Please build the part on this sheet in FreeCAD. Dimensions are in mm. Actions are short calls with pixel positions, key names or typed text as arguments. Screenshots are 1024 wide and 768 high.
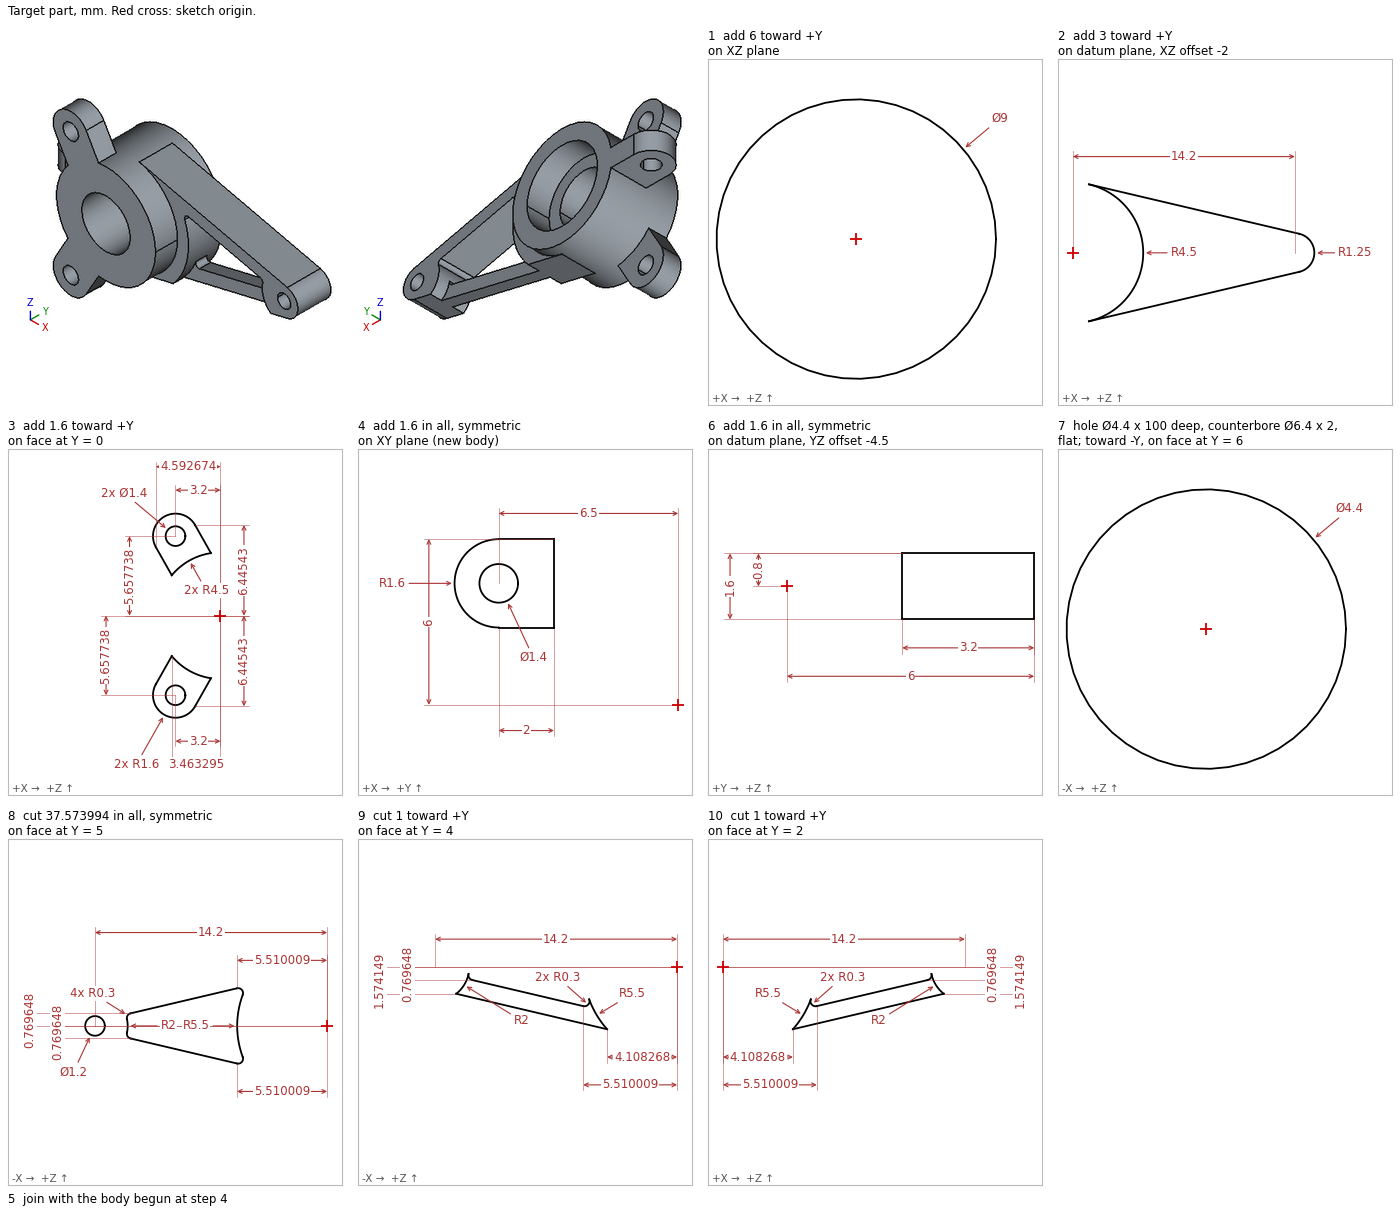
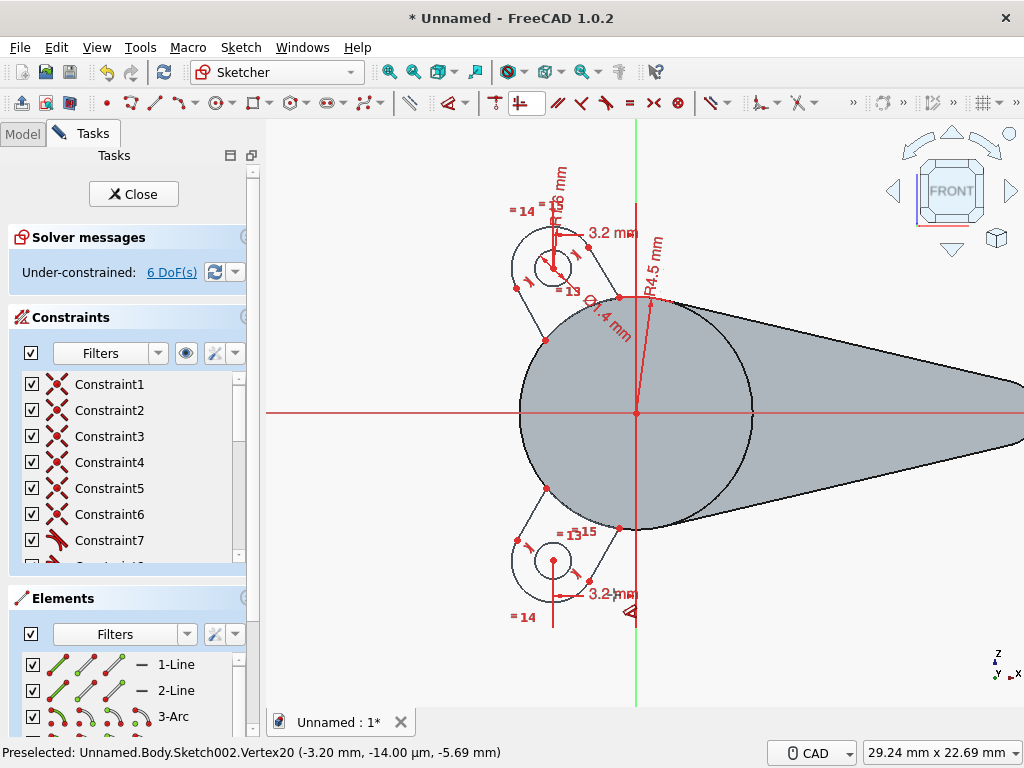
click(589, 247)
click(670, 292)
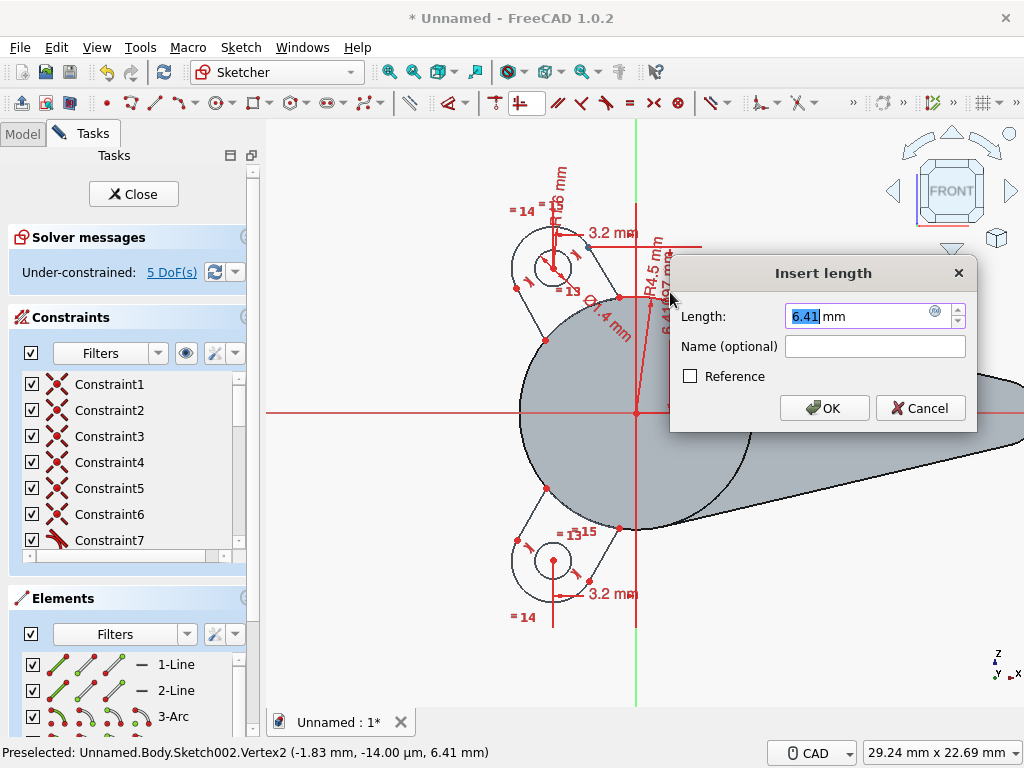
text(6.44543)
key(Return)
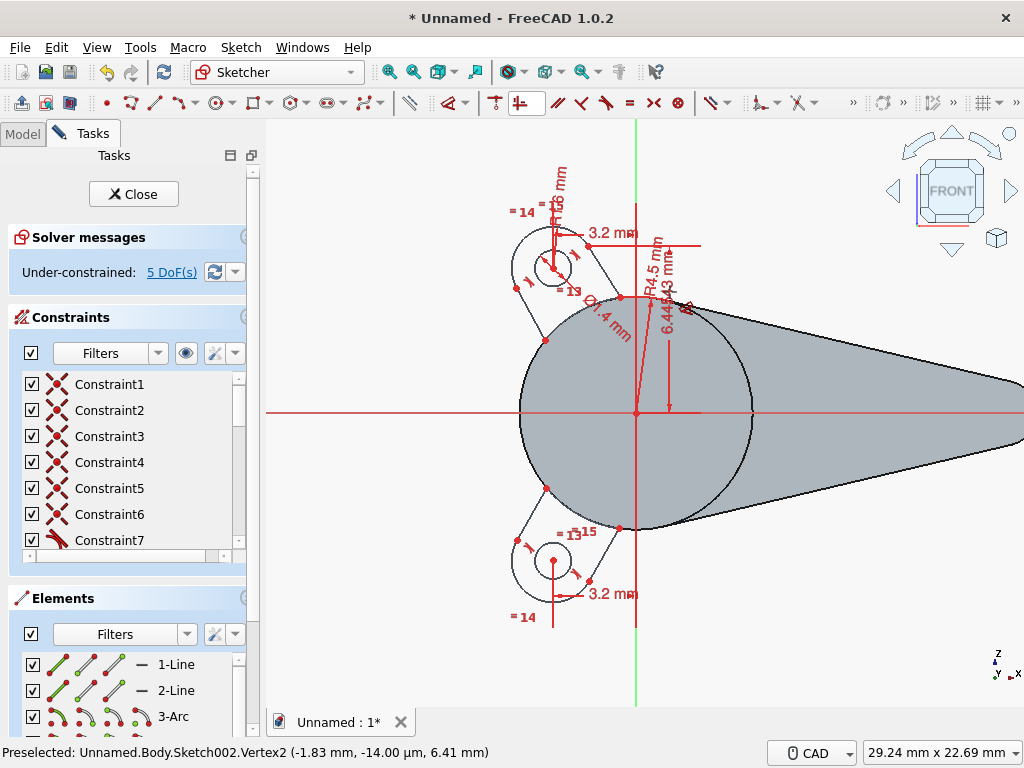
click(589, 581)
click(670, 497)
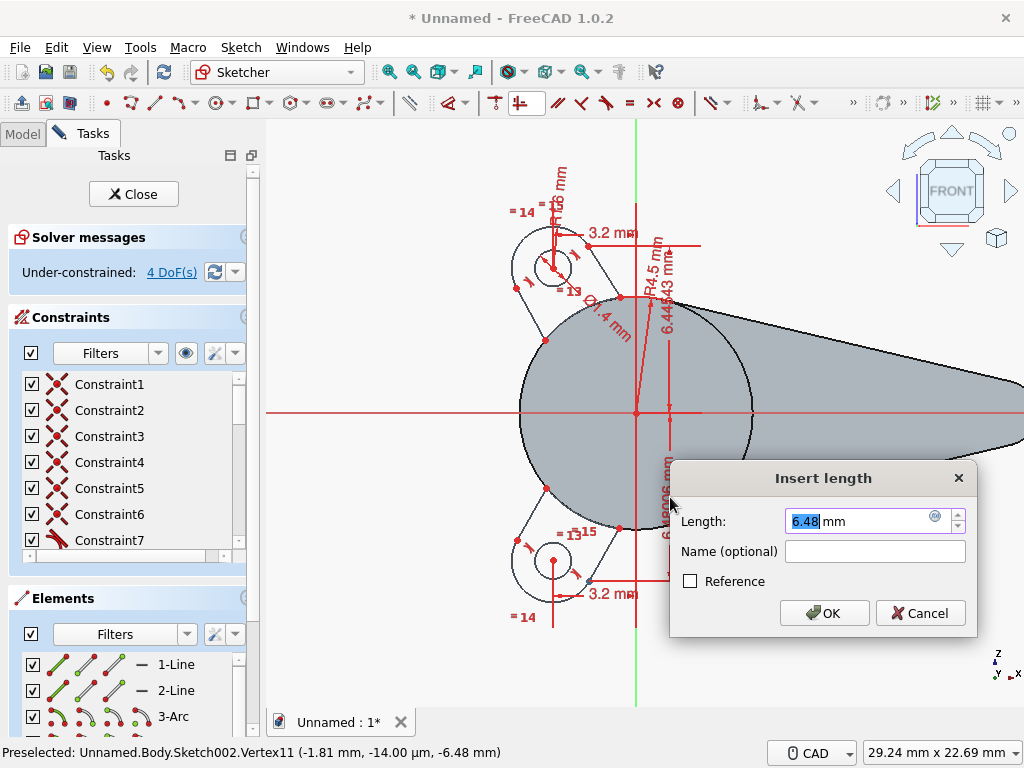
text(6.44543)
key(Return)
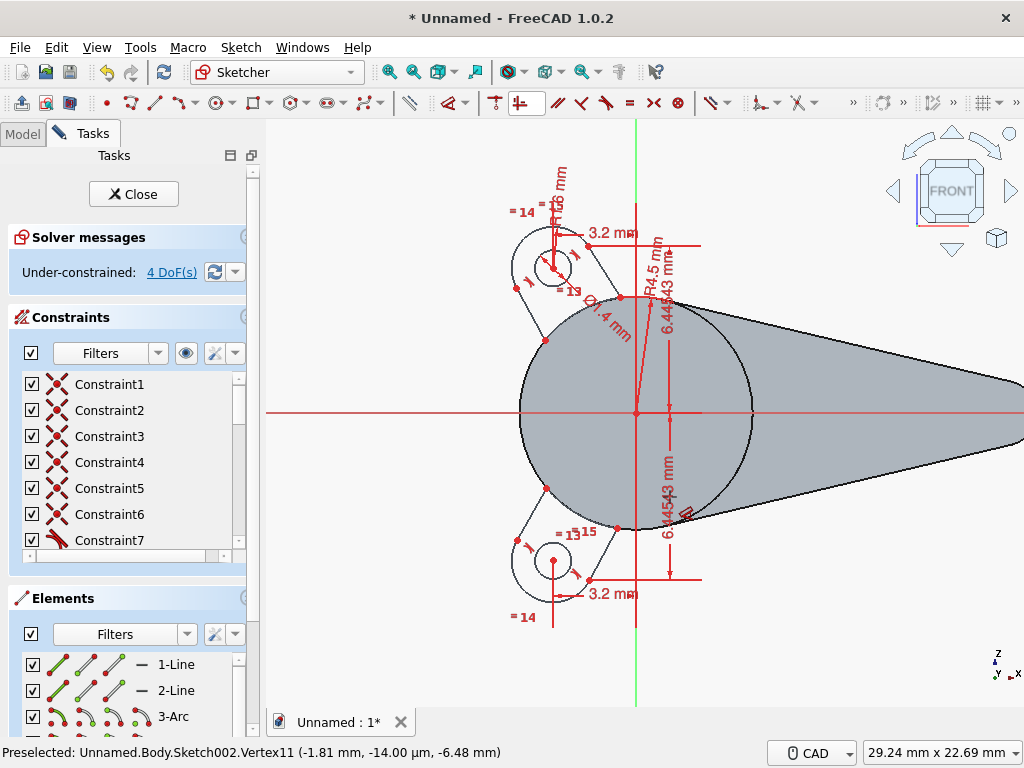
click(553, 268)
click(670, 341)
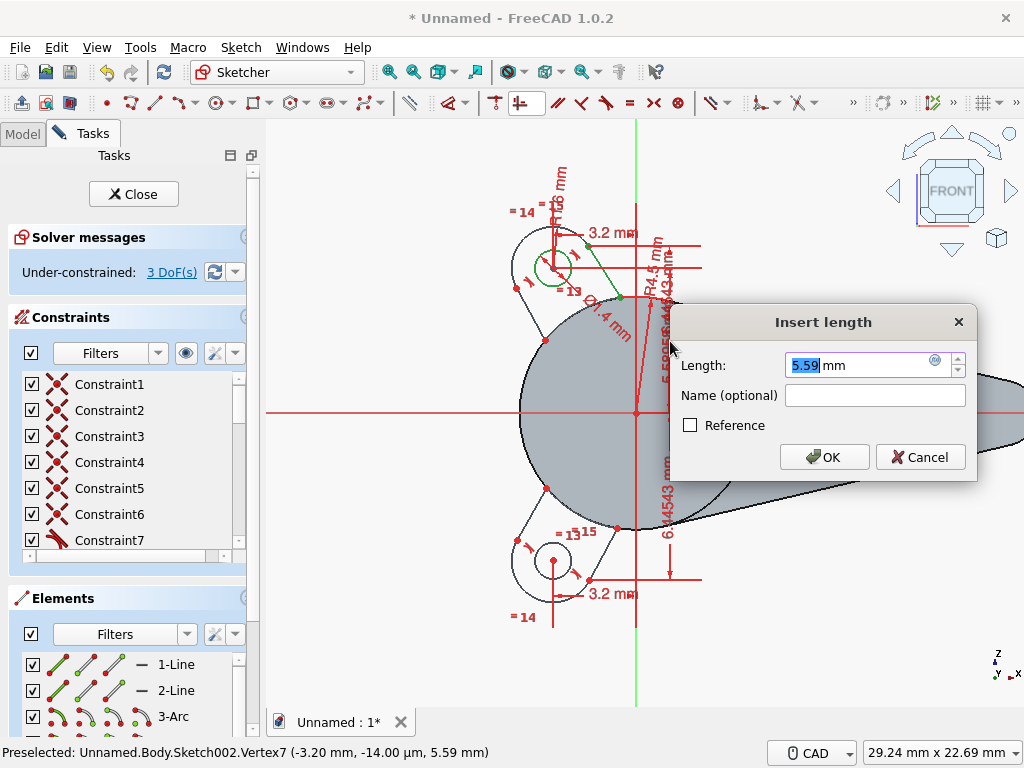
text(5.657738)
key(Return)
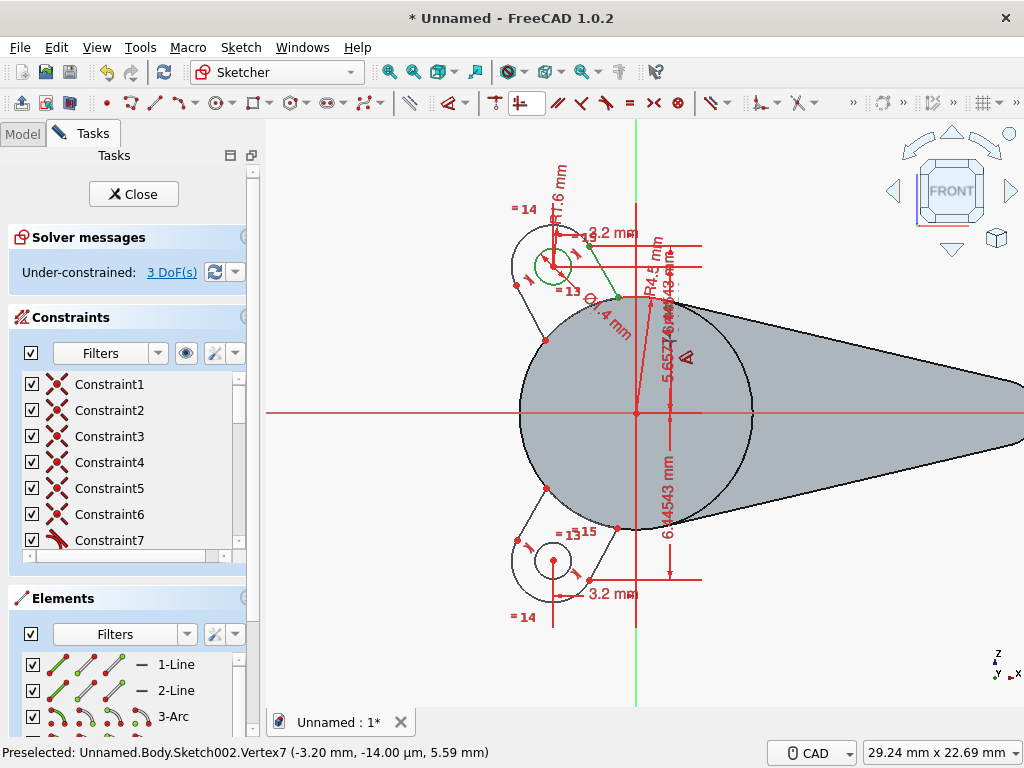
click(553, 561)
click(670, 453)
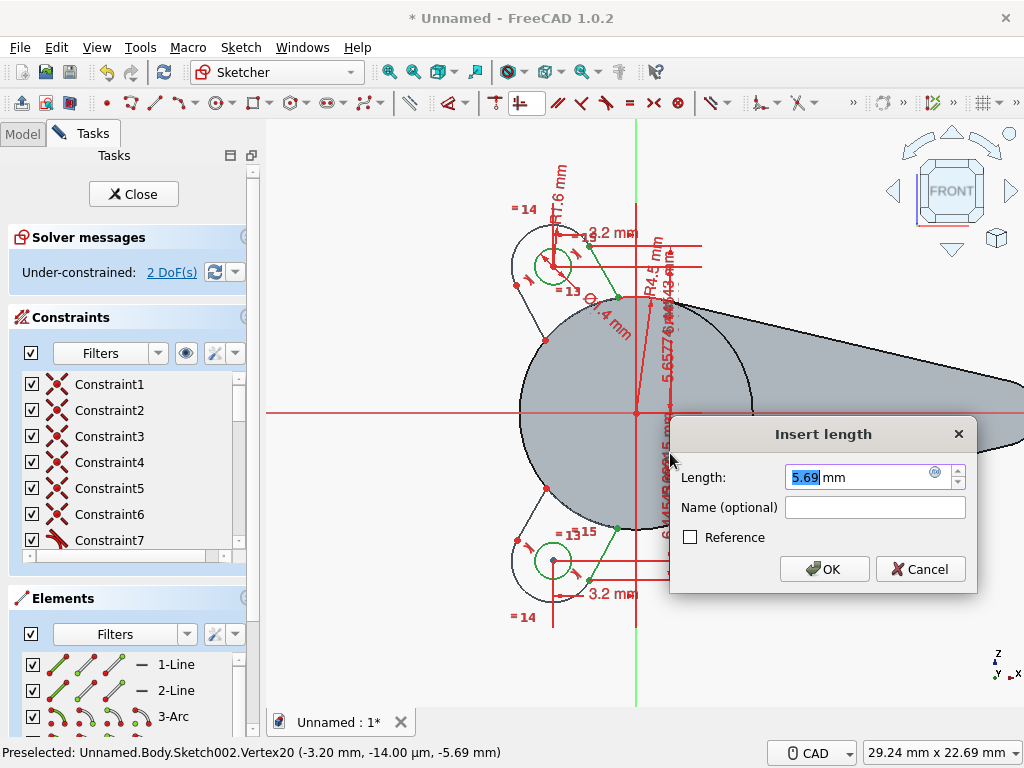
text(5.657738)
key(Return)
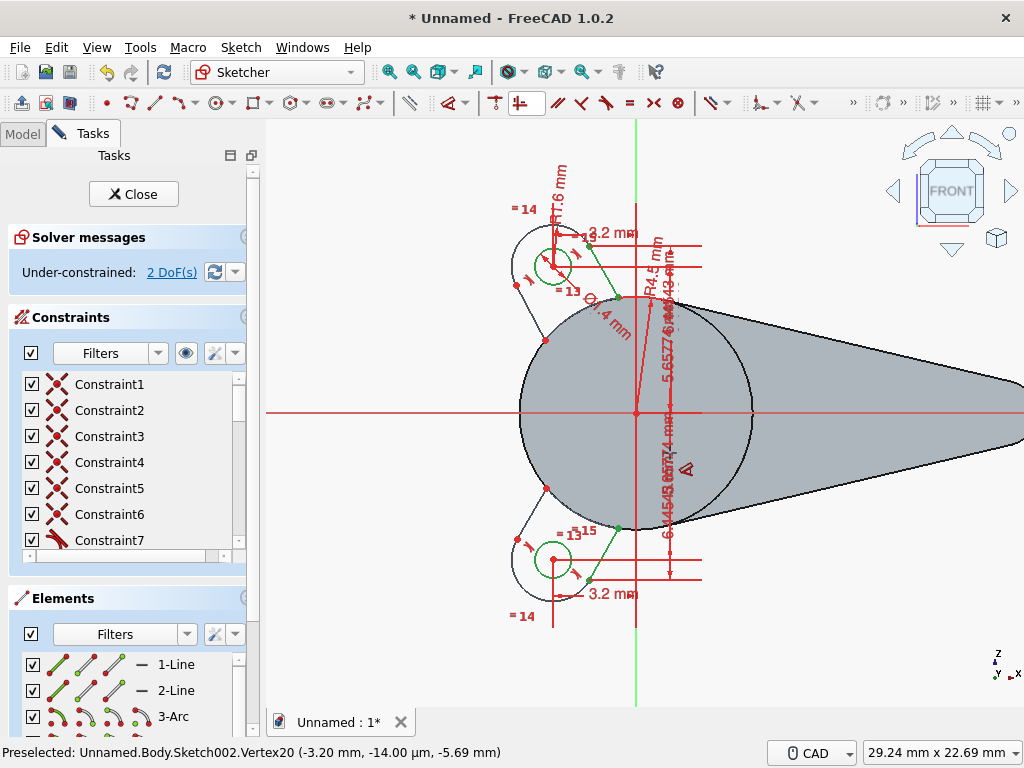
click(516, 286)
click(576, 447)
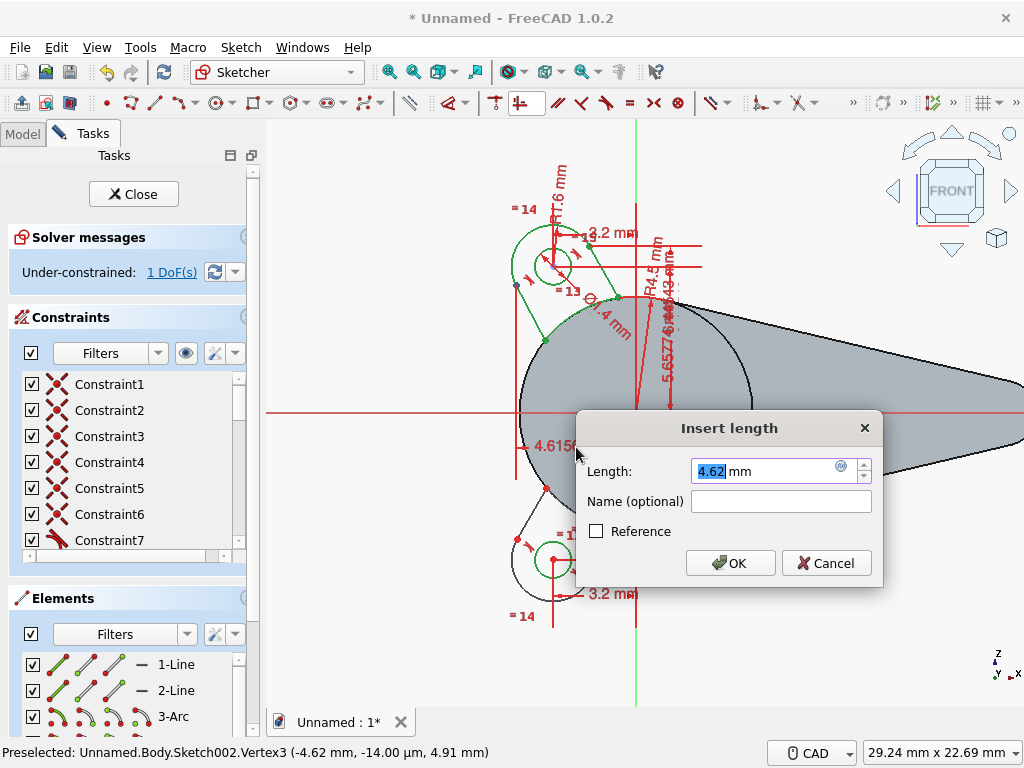
text(4.592674)
key(Return)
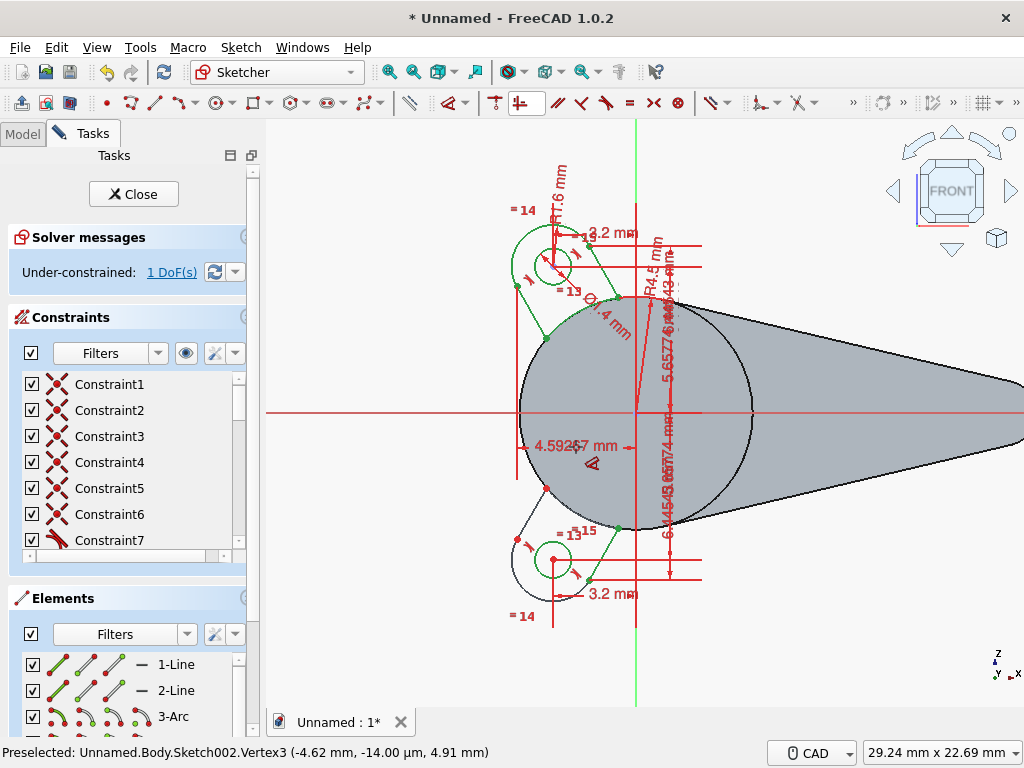
click(547, 488)
click(560, 522)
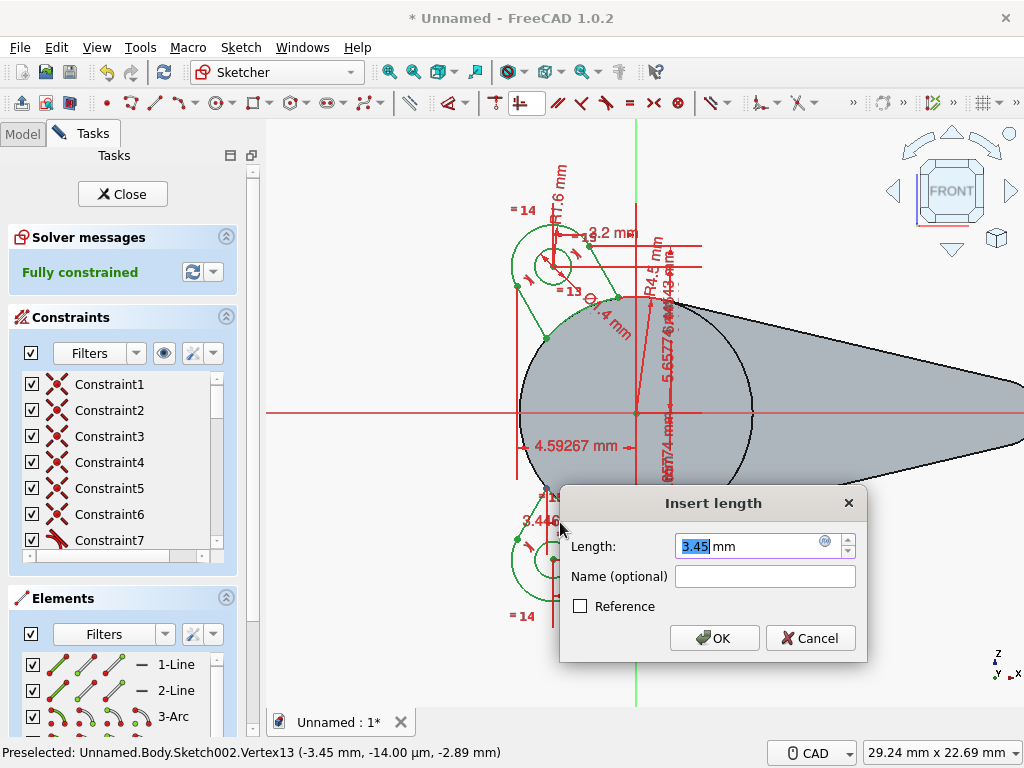
text(3.463295)
key(Return)
key(Escape)